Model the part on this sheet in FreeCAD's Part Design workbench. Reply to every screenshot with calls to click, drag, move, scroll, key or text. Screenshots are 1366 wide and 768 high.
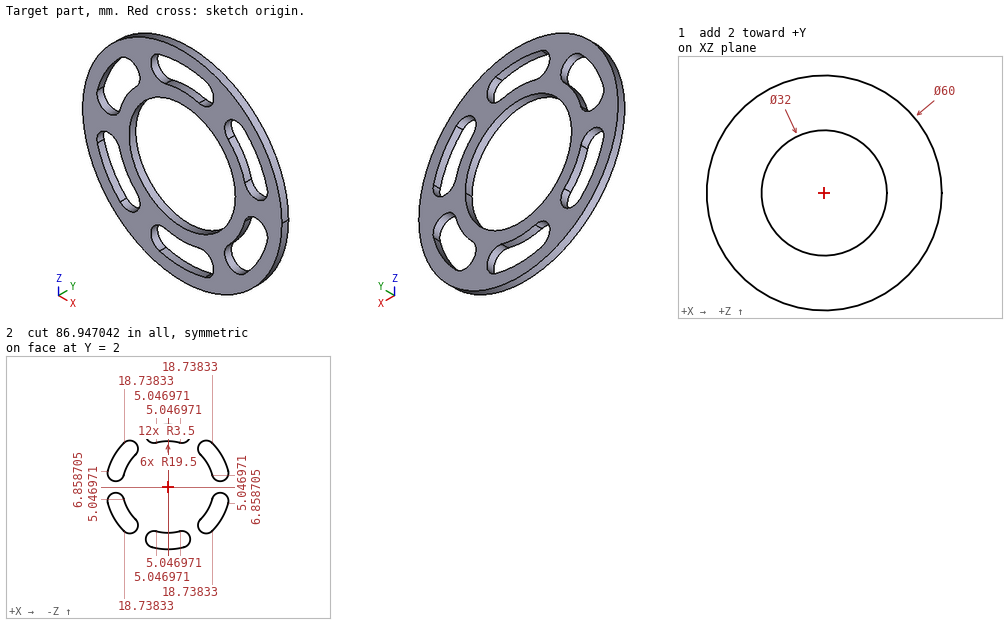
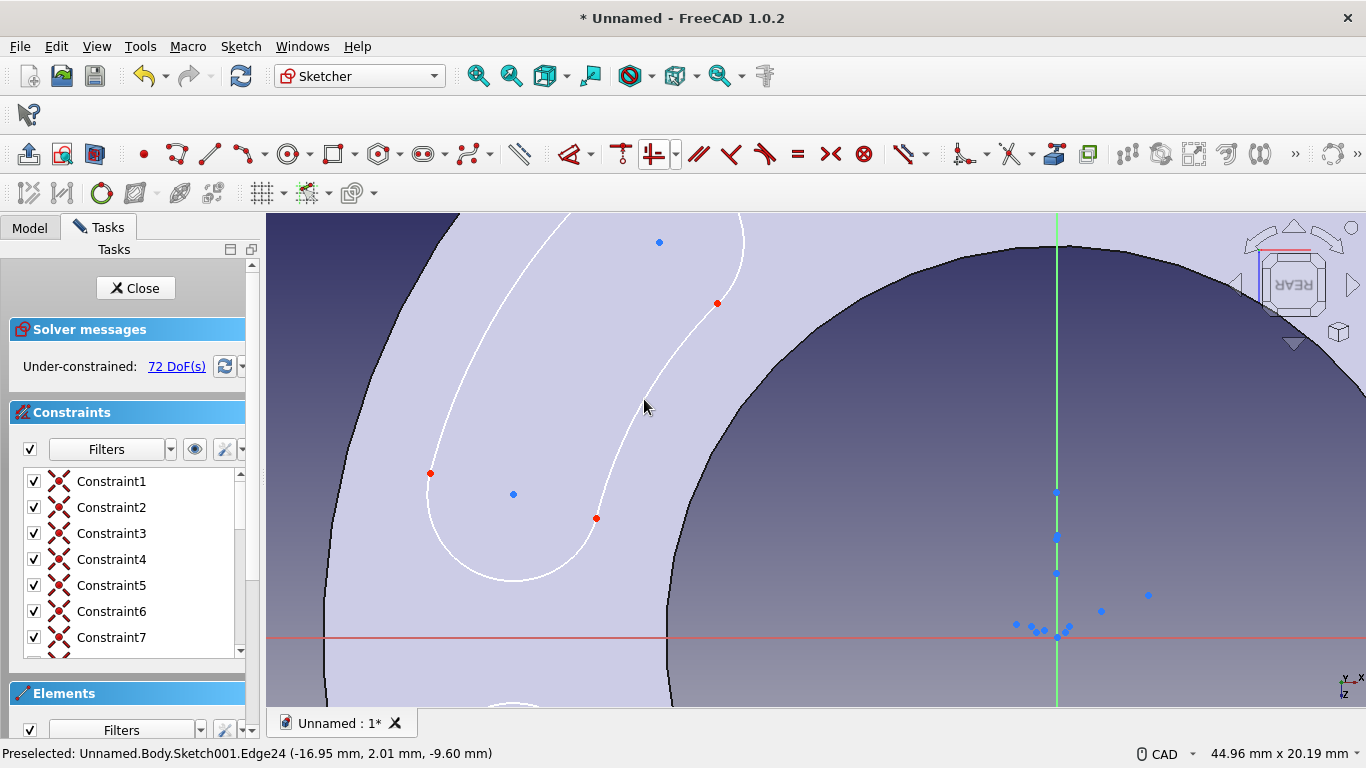
scroll(646, 402, down, 7)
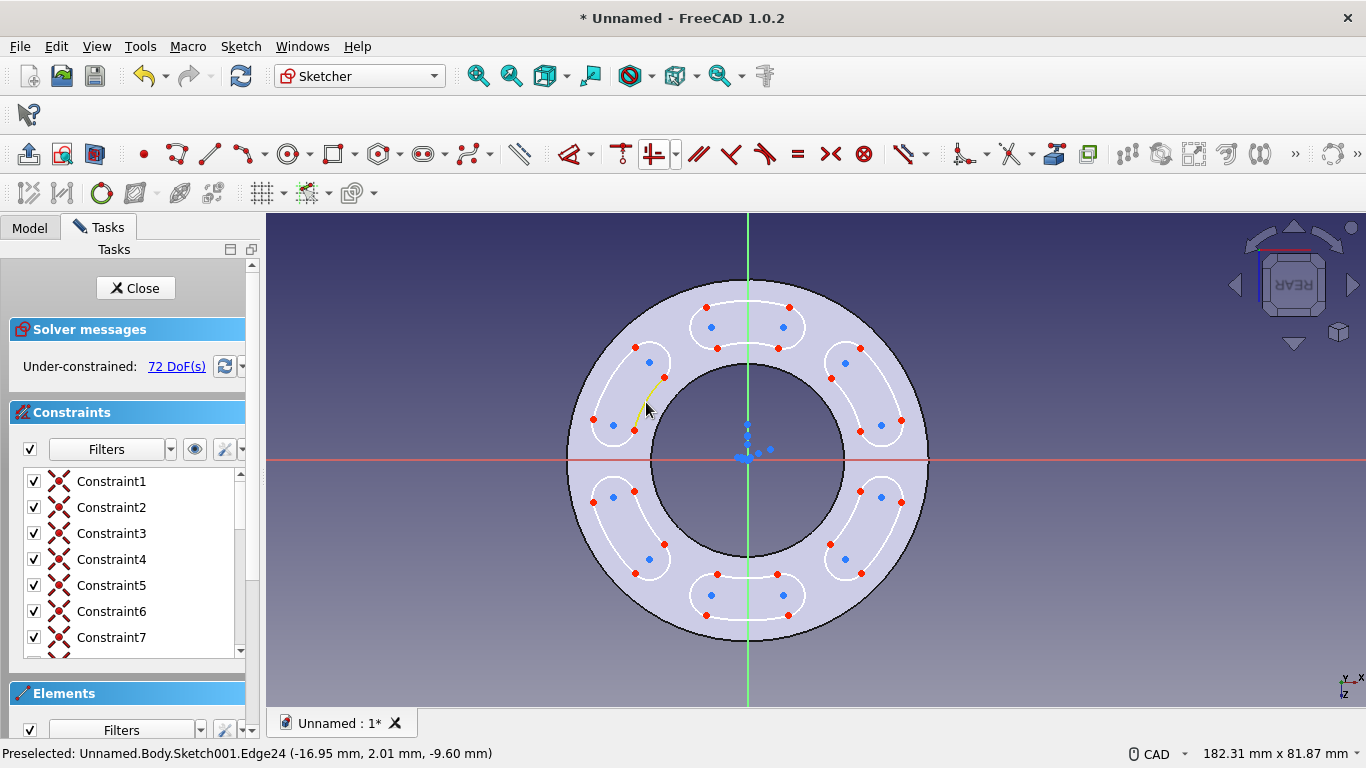
click(760, 344)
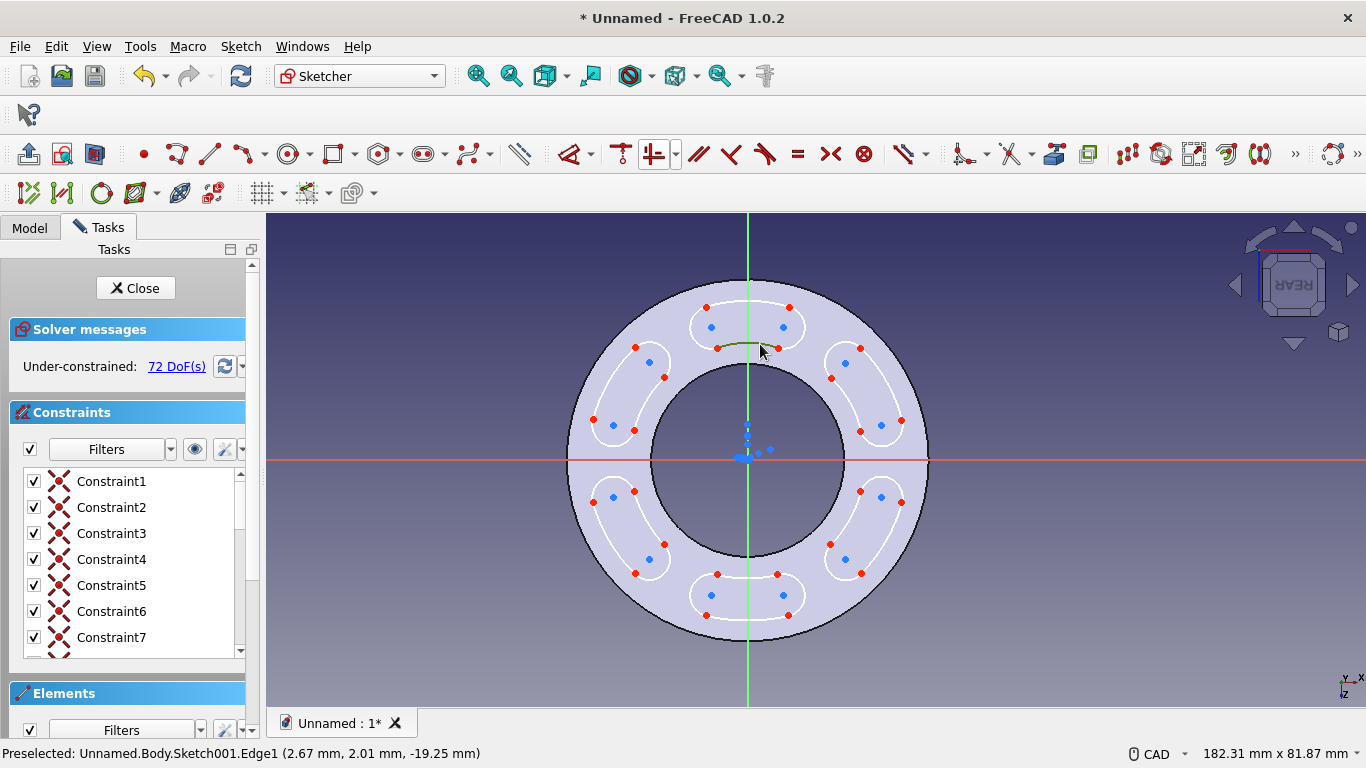
click(797, 344)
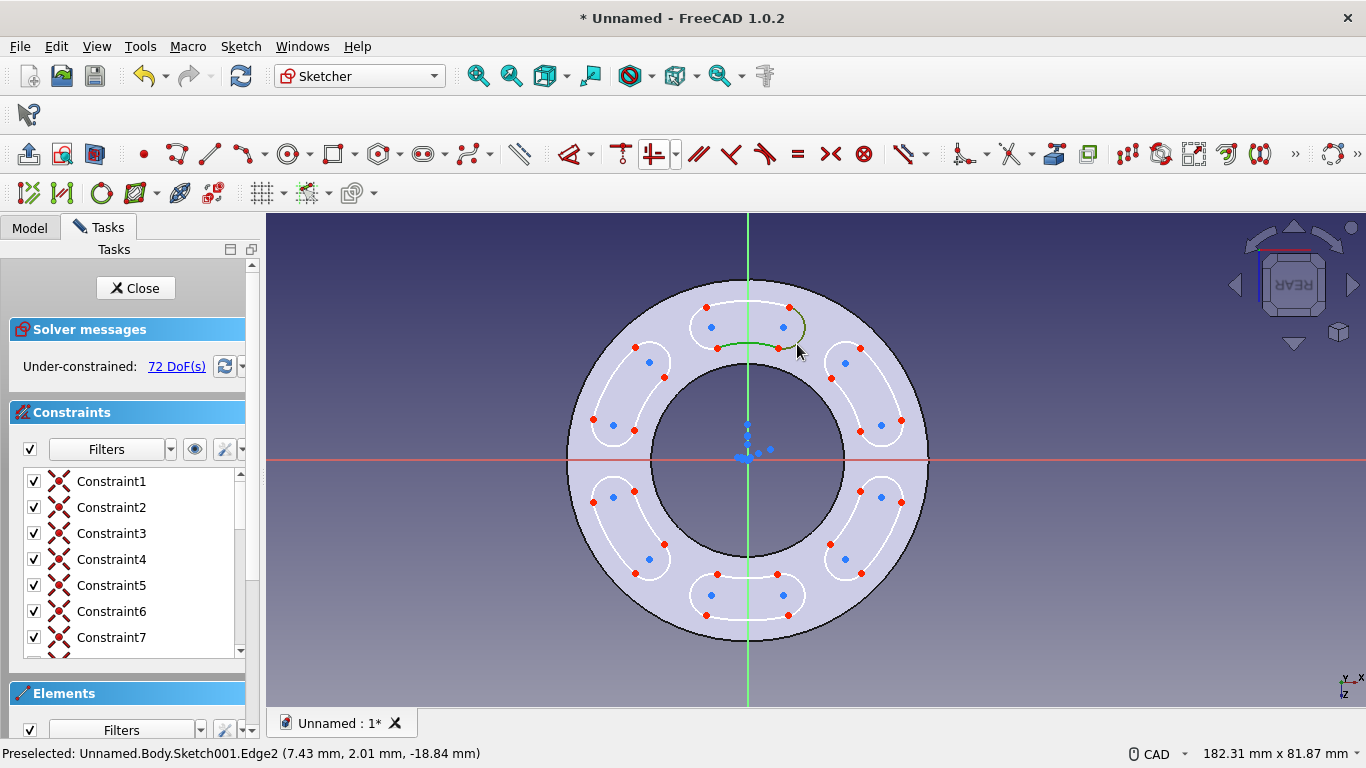
key(t)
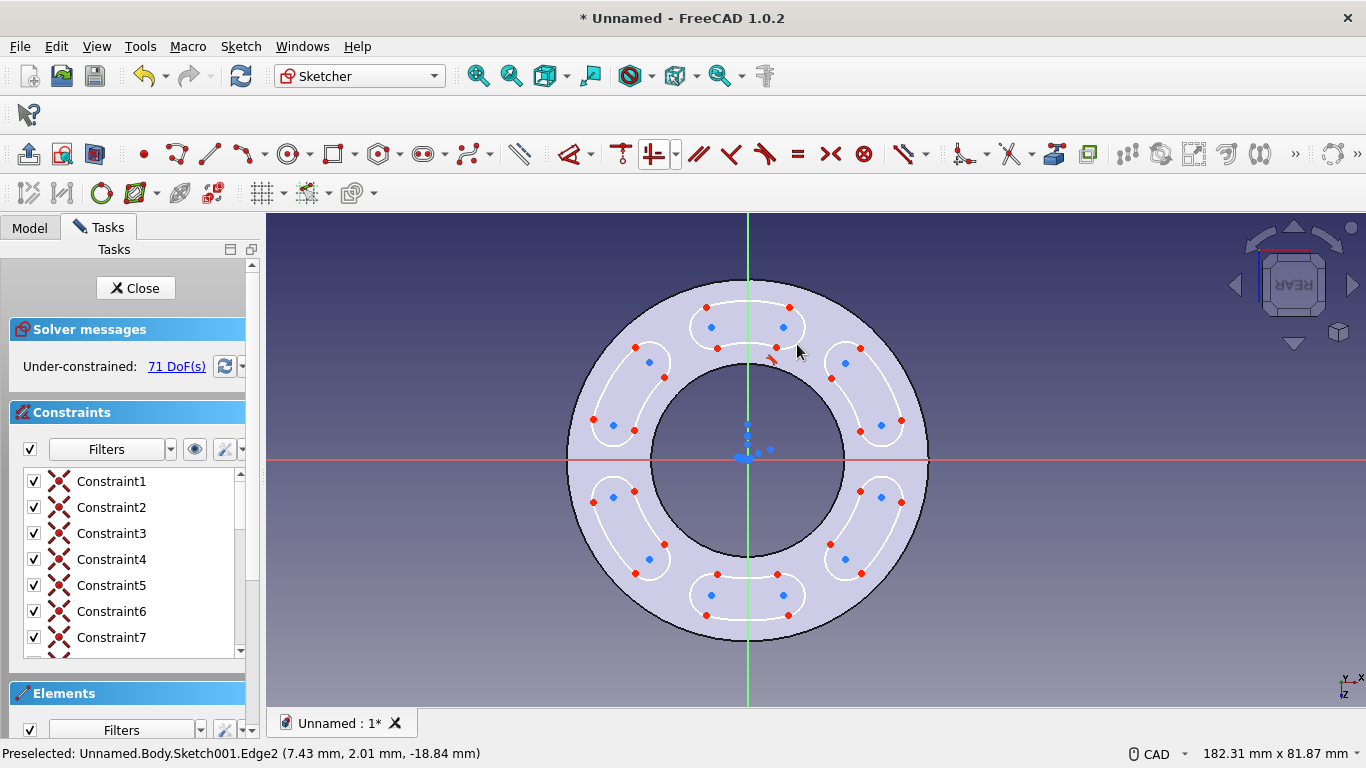
click(759, 344)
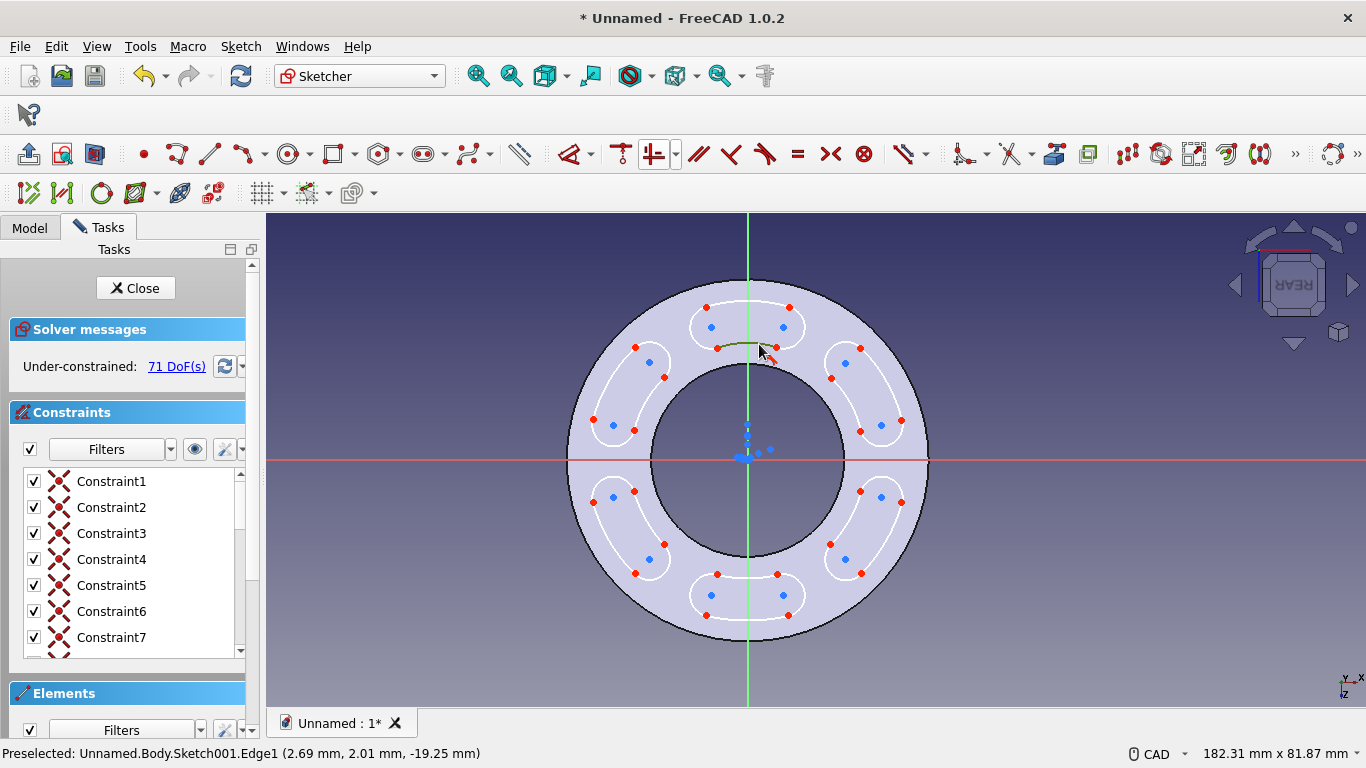
click(692, 320)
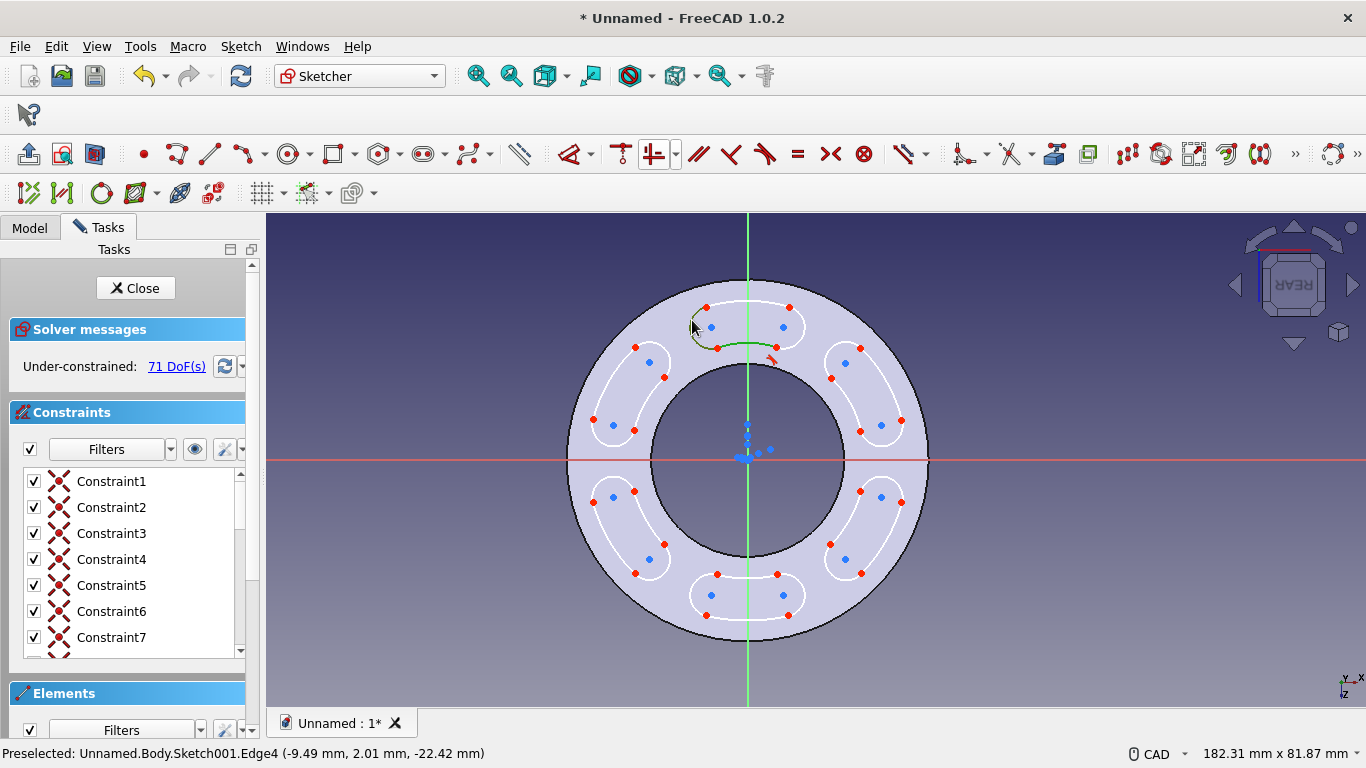
click(765, 154)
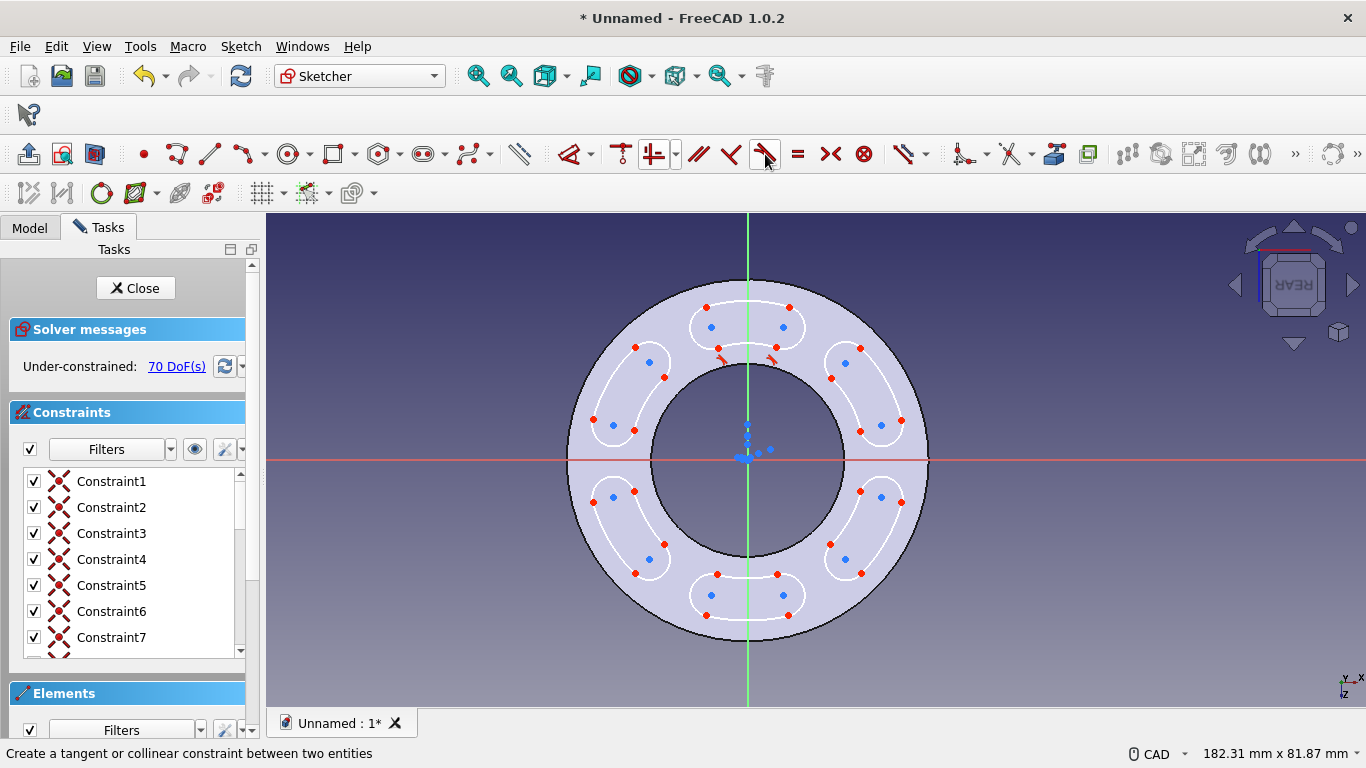
click(796, 345)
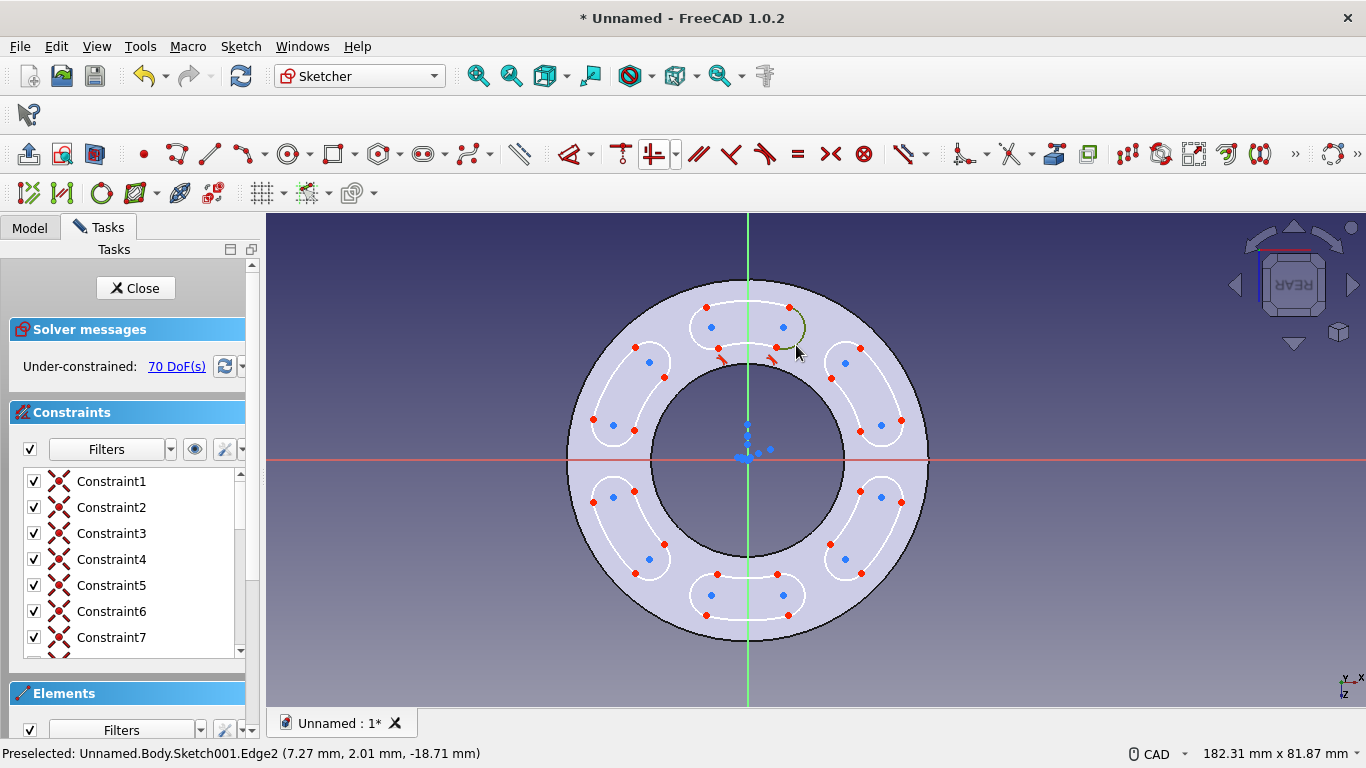
click(764, 302)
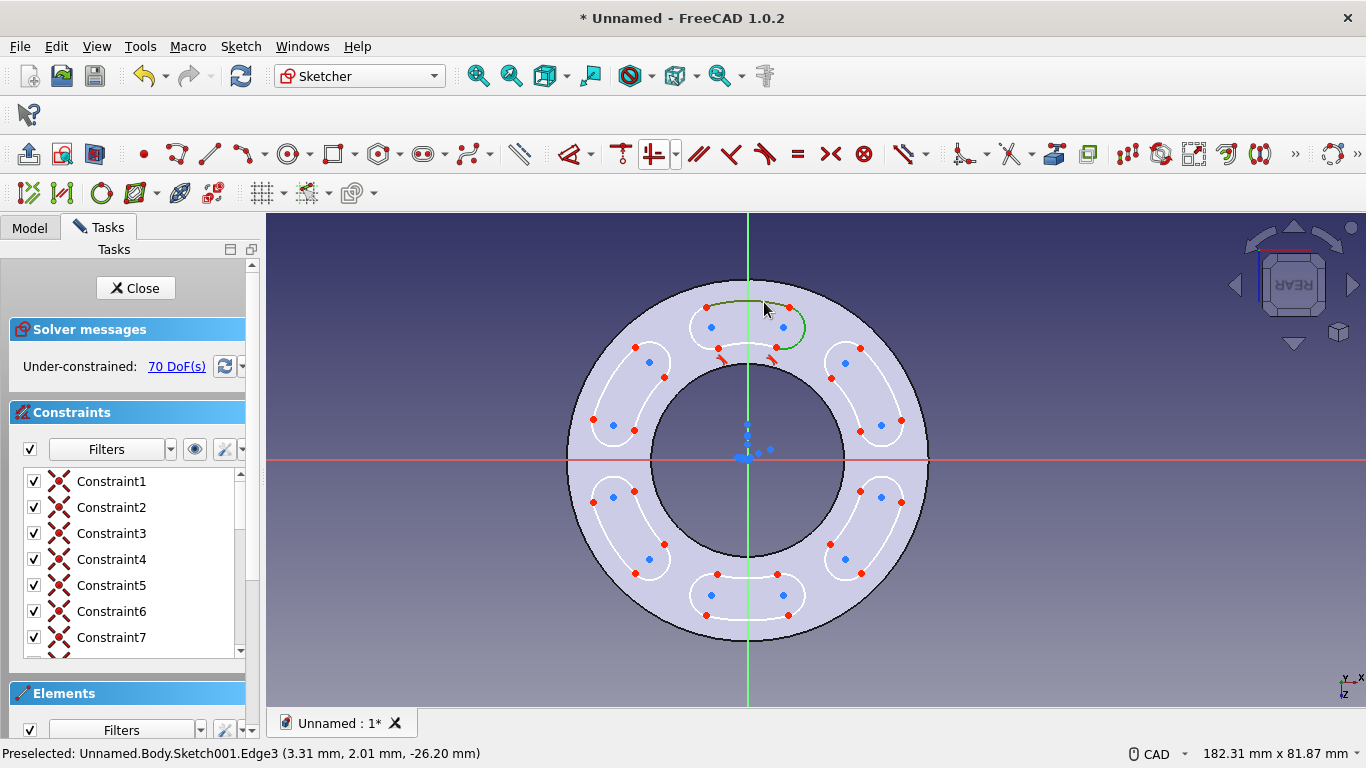
key(t)